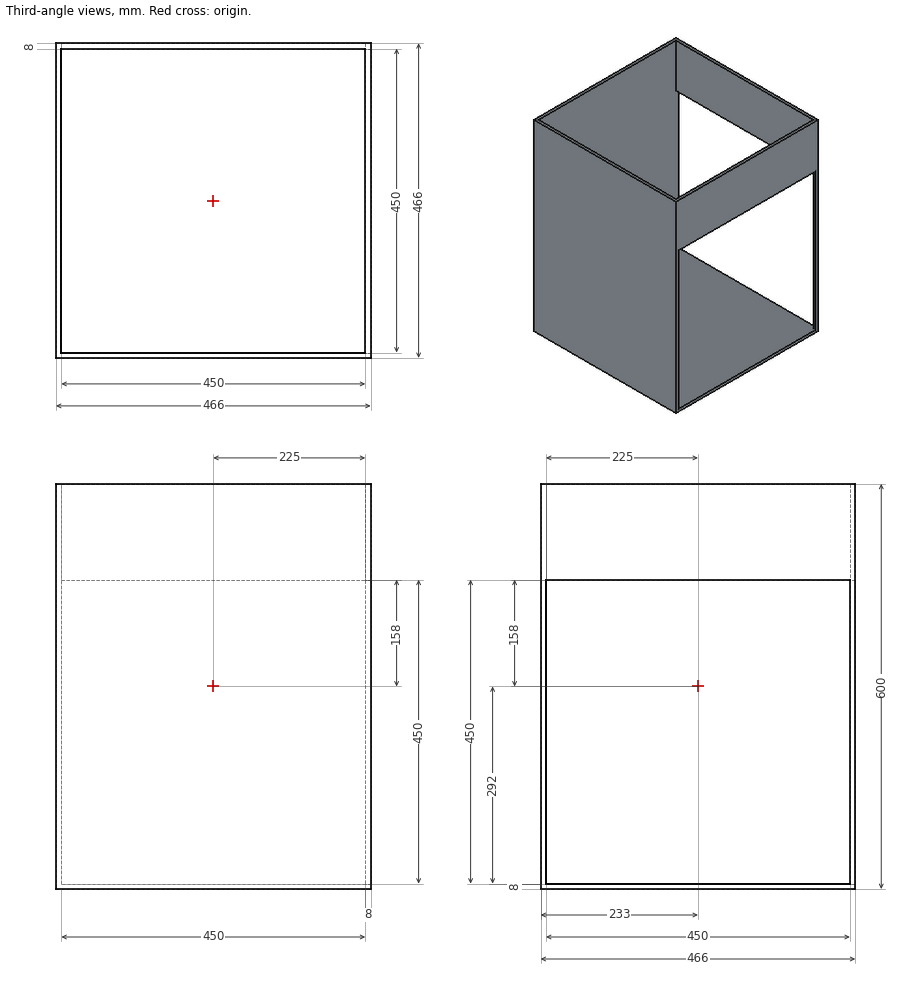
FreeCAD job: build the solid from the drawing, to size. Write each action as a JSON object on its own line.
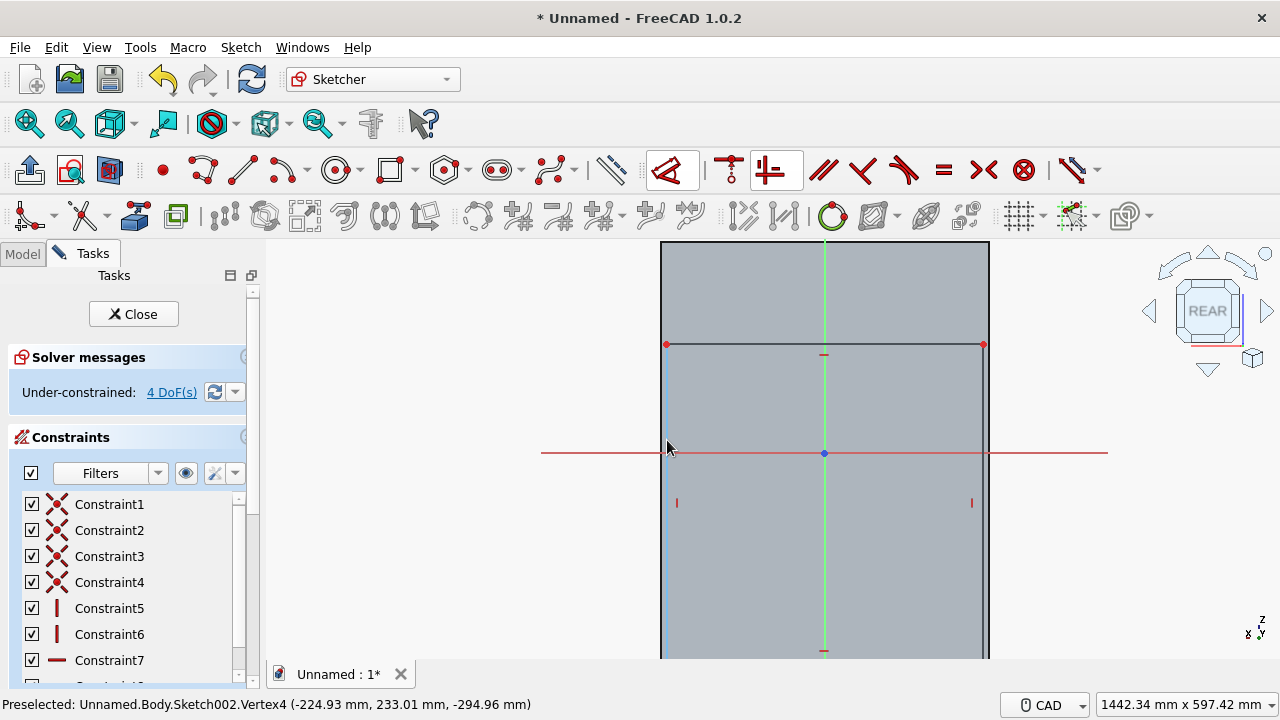
{"action": "left_click", "coordinate": [667, 439]}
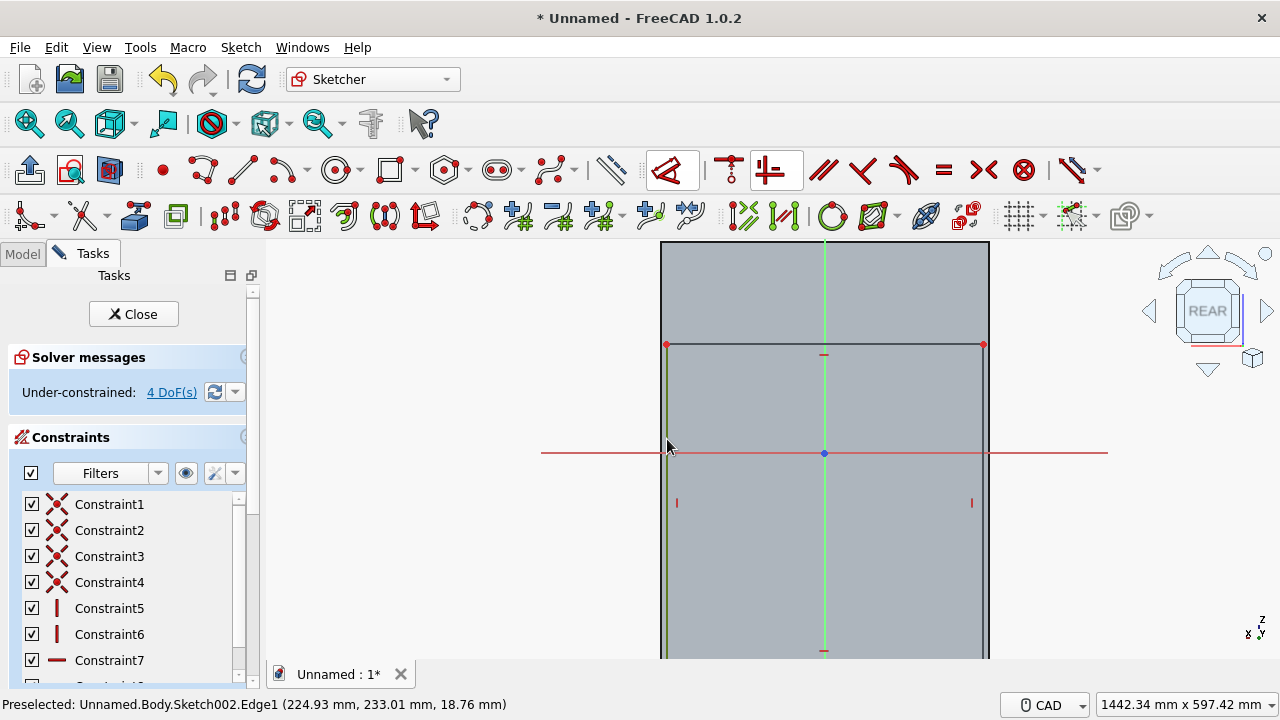
{"action": "key", "text": "i"}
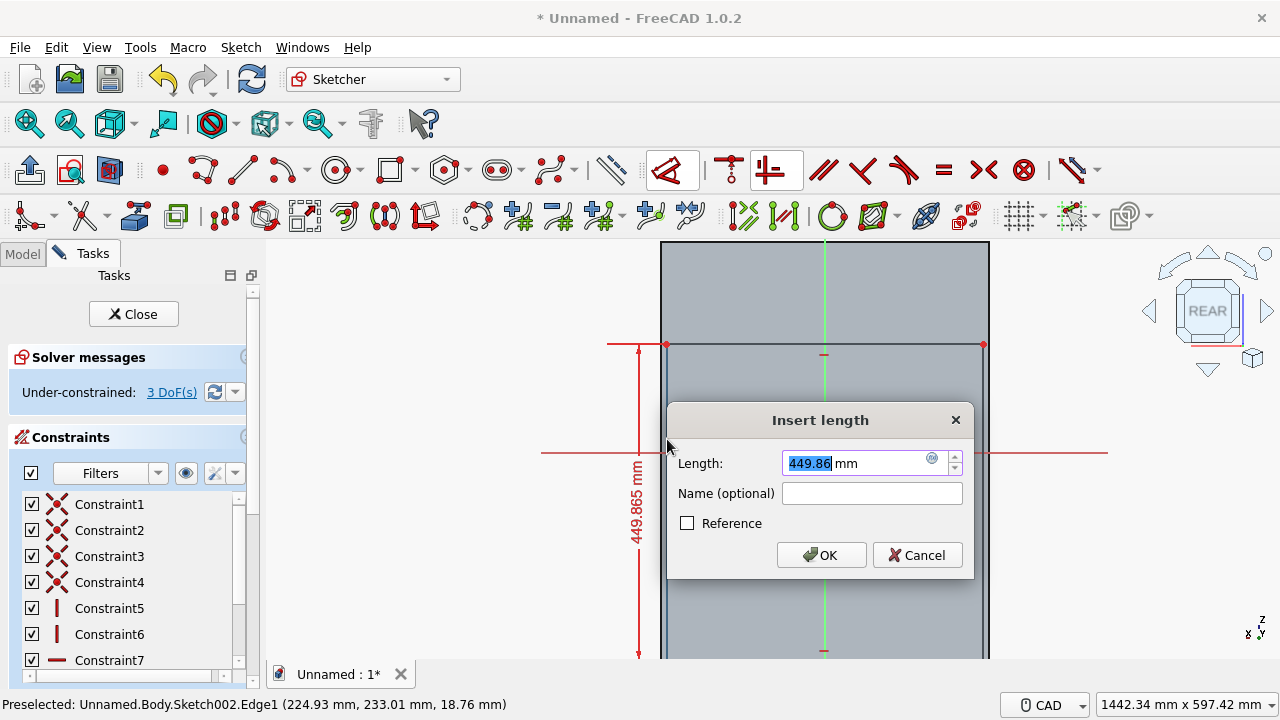
{"action": "type", "text": "450"}
{"action": "key", "text": "Return"}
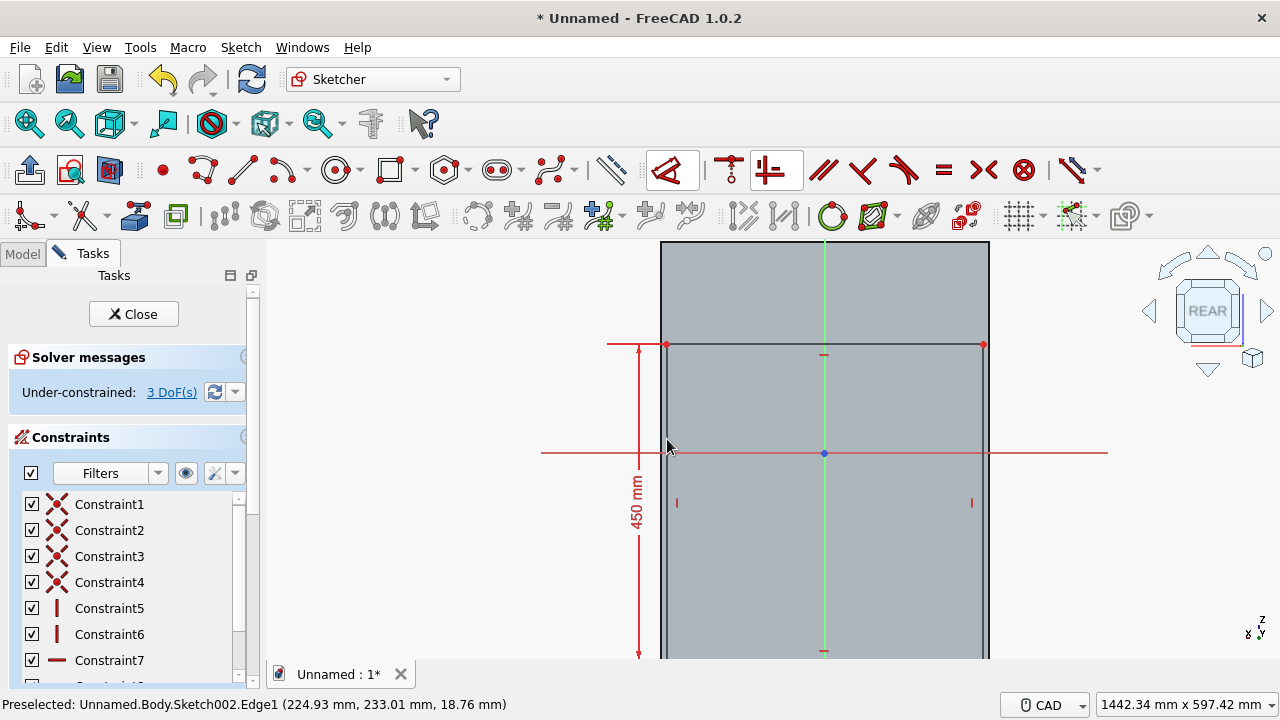
{"action": "scroll", "coordinate": [294, 267], "scroll_direction": "down", "scroll_amount": 1}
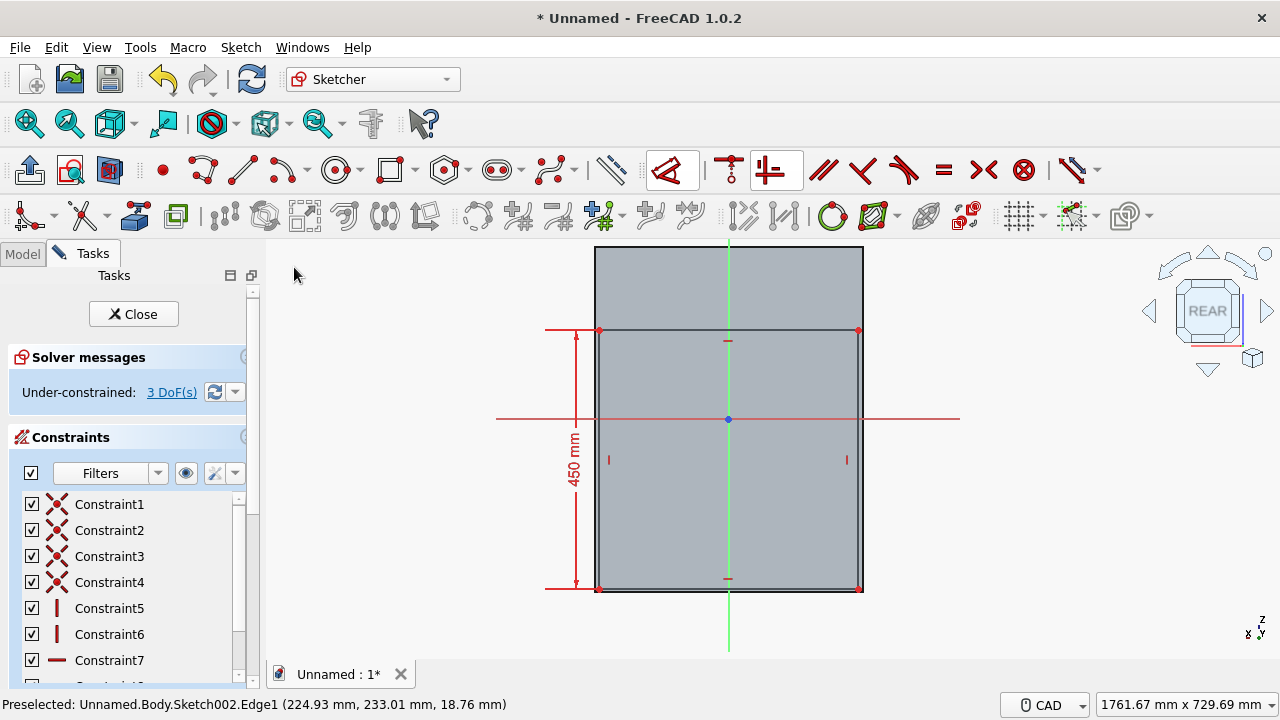
{"action": "left_click", "coordinate": [677, 589]}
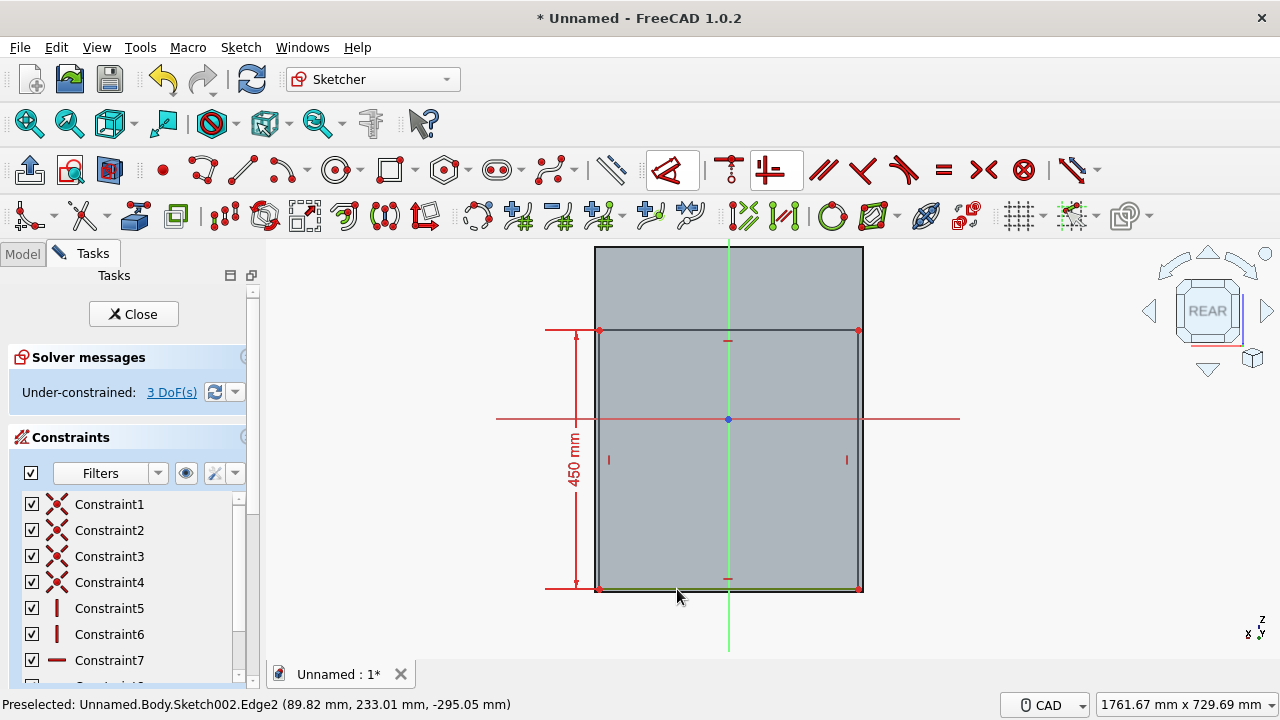
{"action": "left_click", "coordinate": [694, 170]}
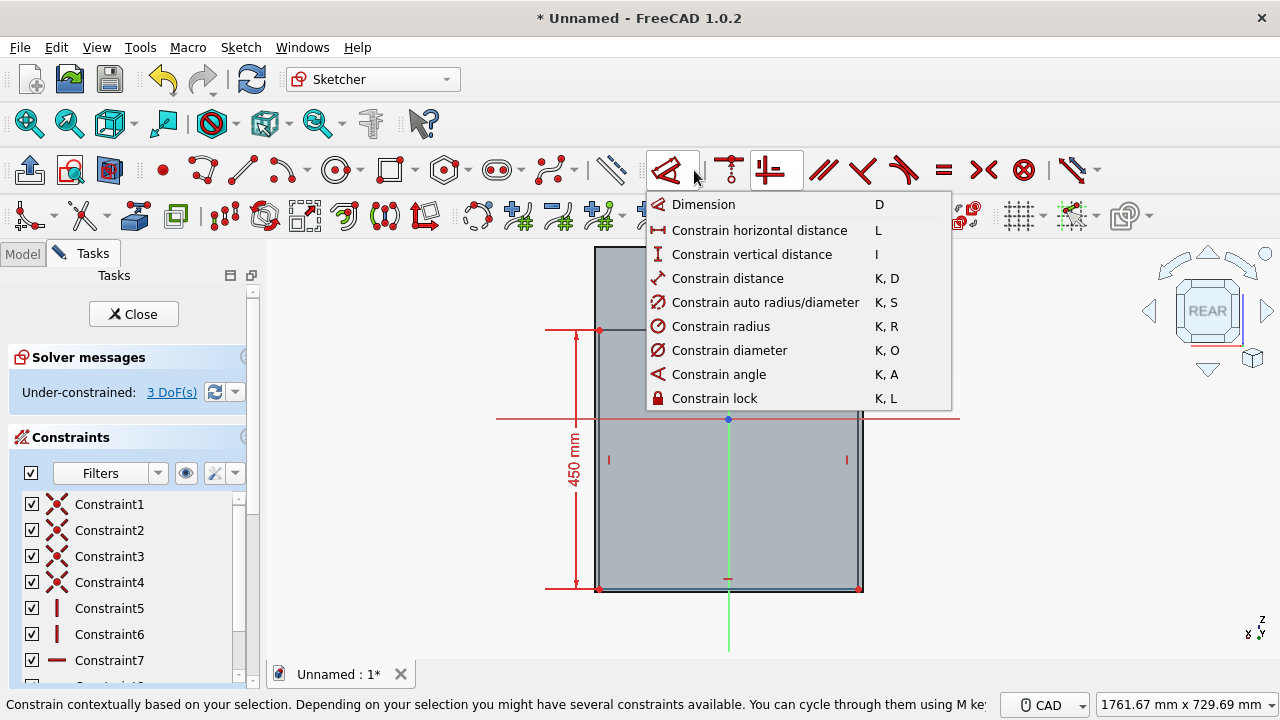
{"action": "left_click", "coordinate": [799, 230]}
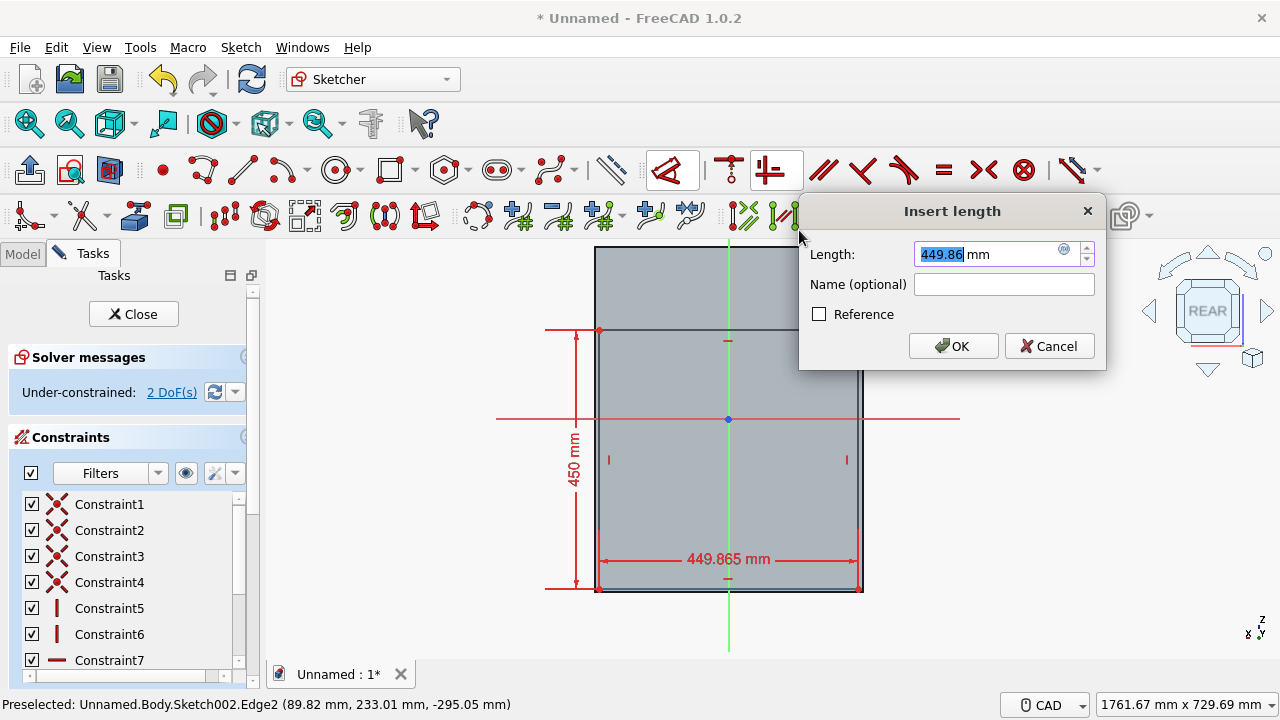
{"action": "type", "text": "450"}
{"action": "key", "text": "Return"}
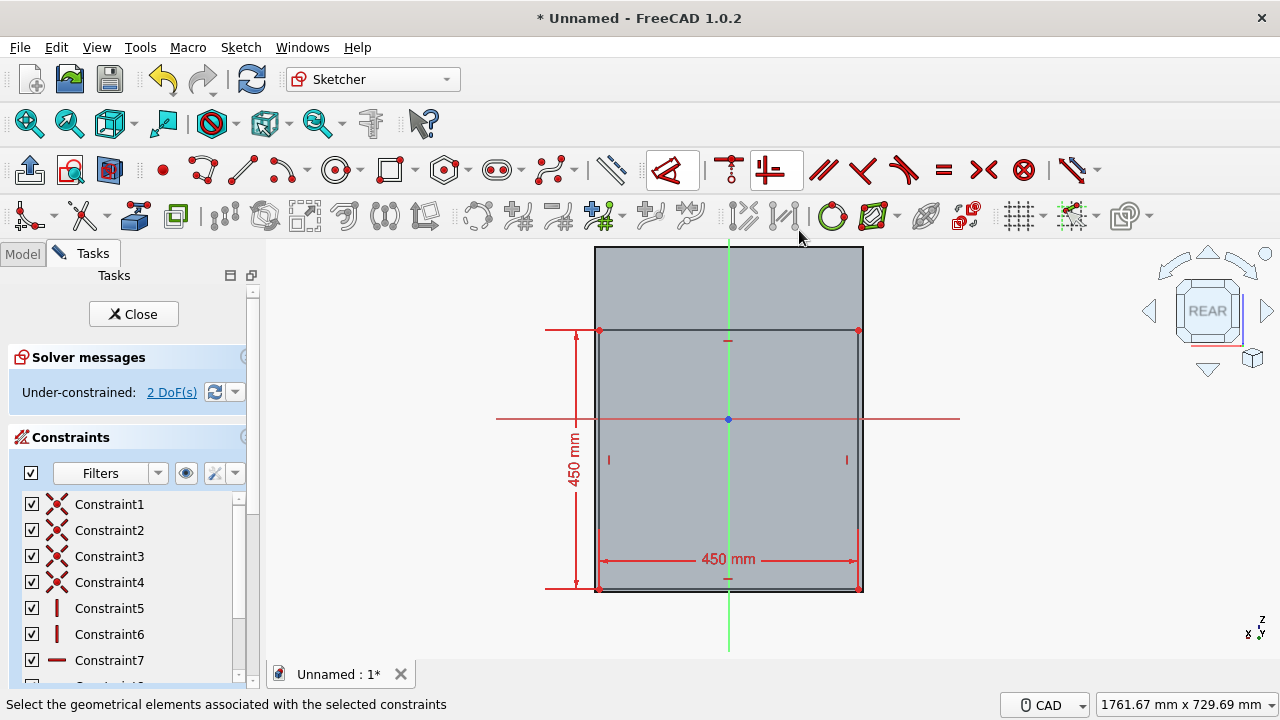
{"action": "left_click", "coordinate": [599, 330]}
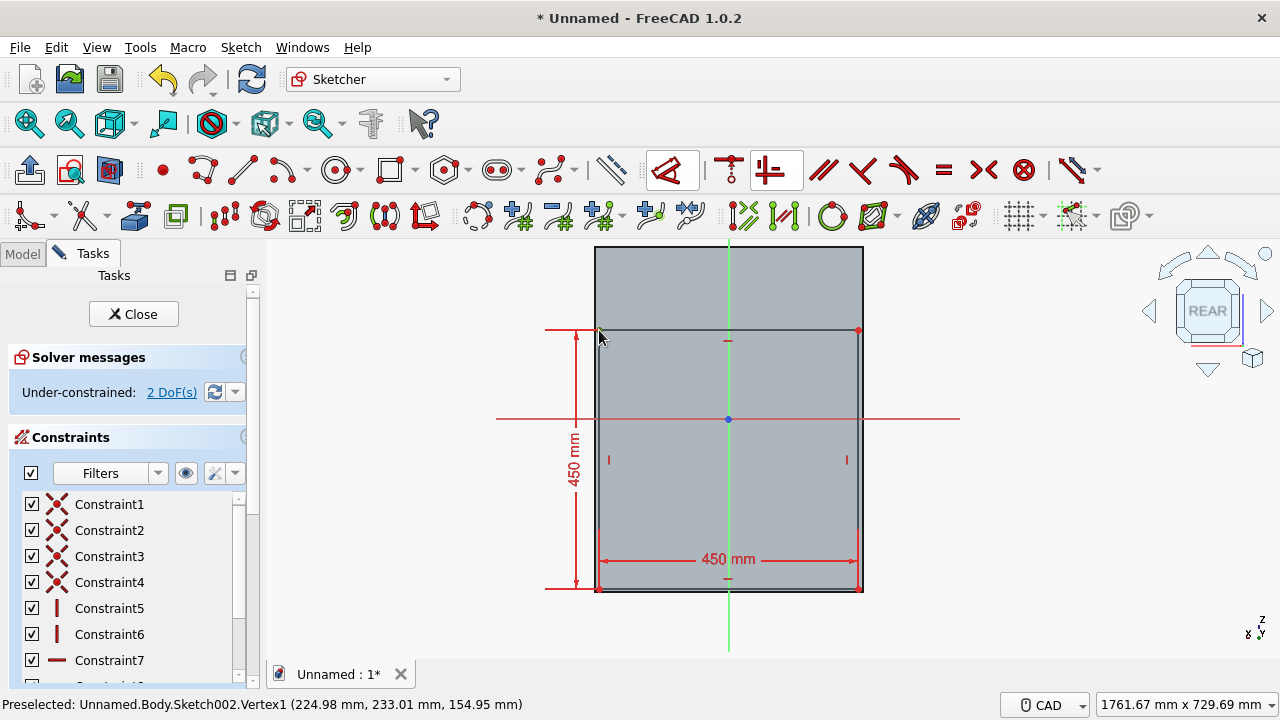
{"action": "left_click", "coordinate": [694, 170]}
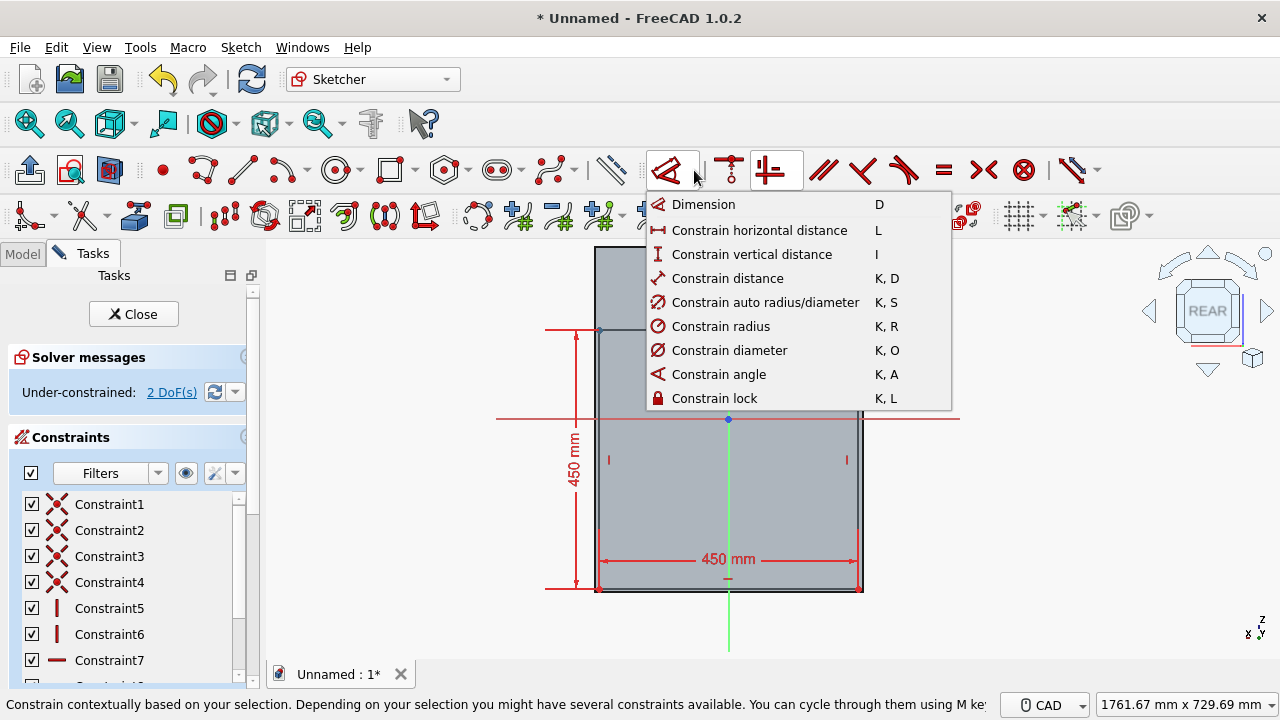
{"action": "left_click", "coordinate": [799, 230]}